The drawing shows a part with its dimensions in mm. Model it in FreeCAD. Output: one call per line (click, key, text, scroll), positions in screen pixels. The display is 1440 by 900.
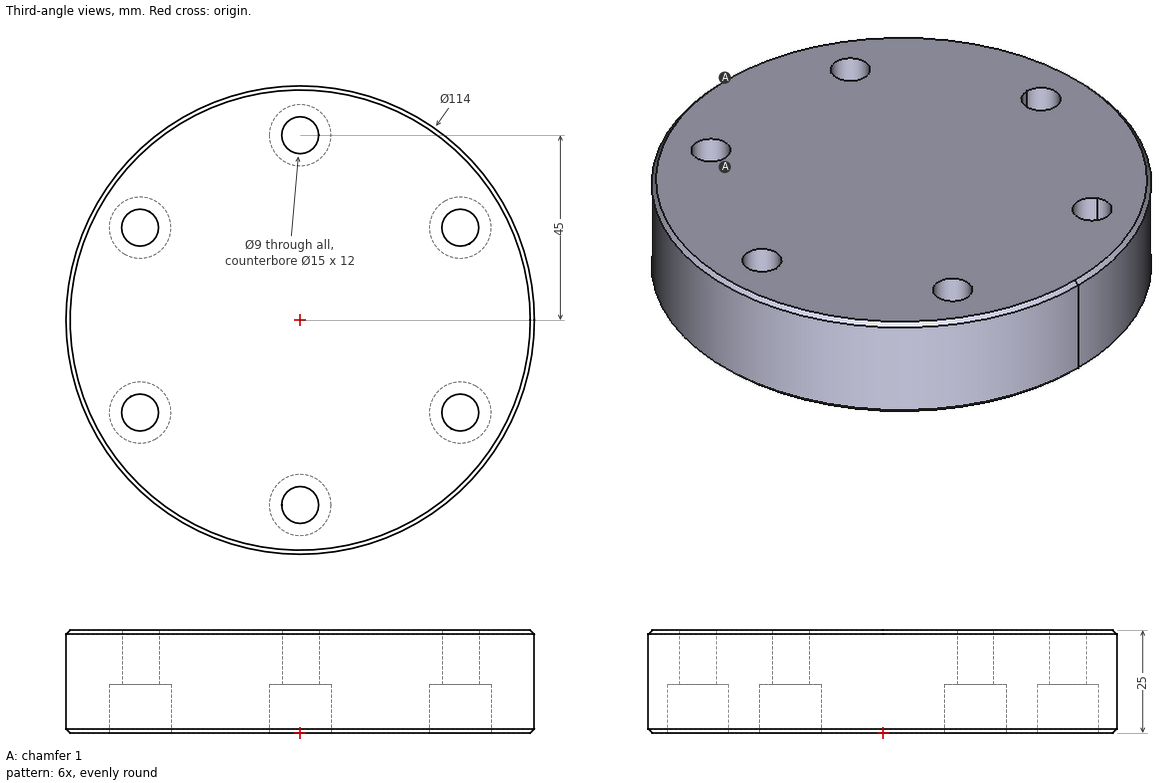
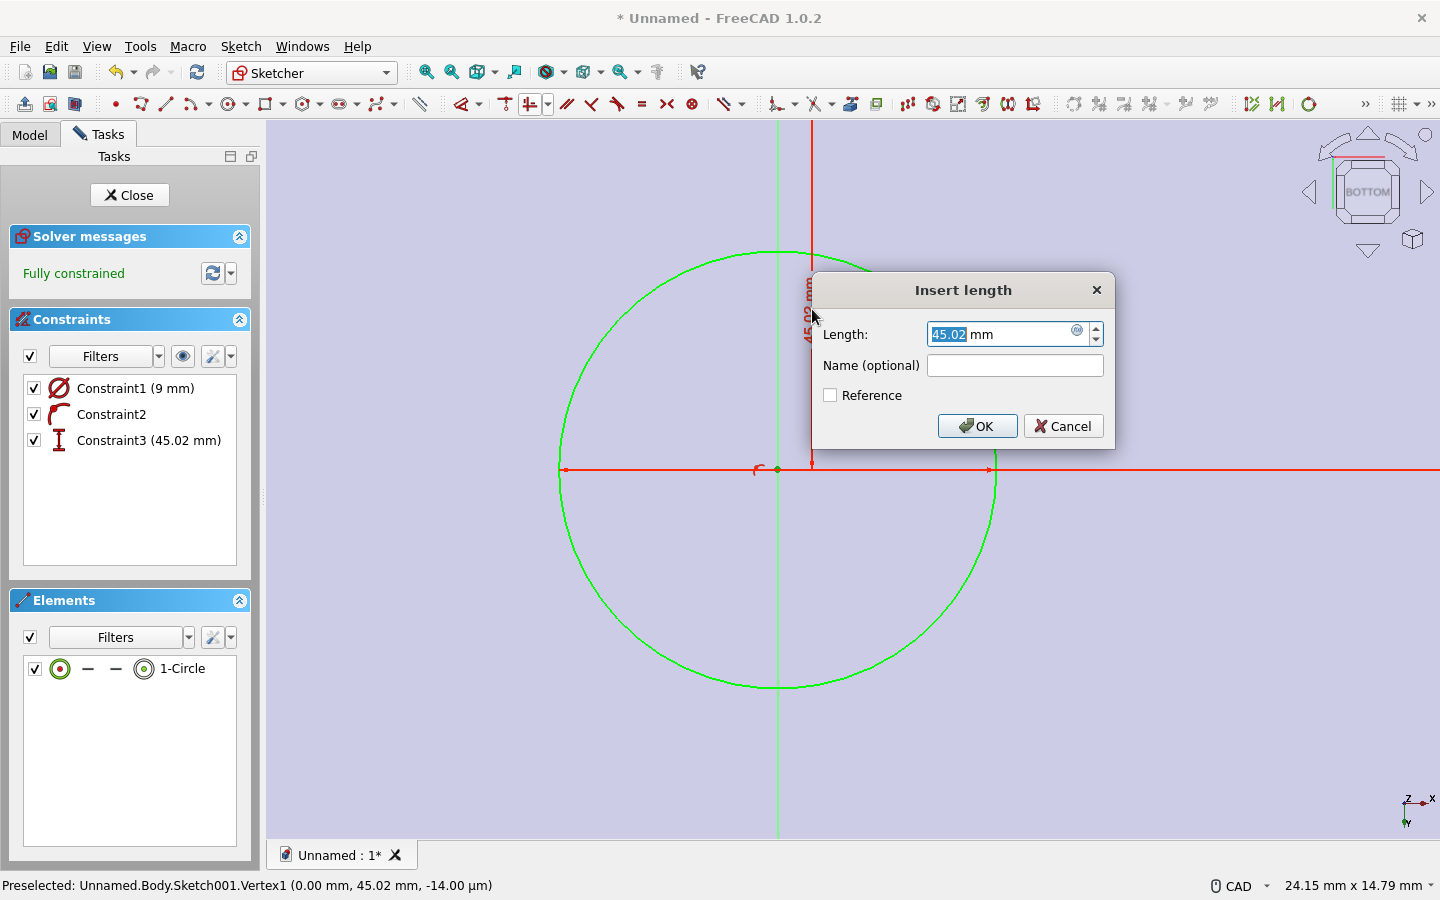
text(45)
key(Return)
key(Escape)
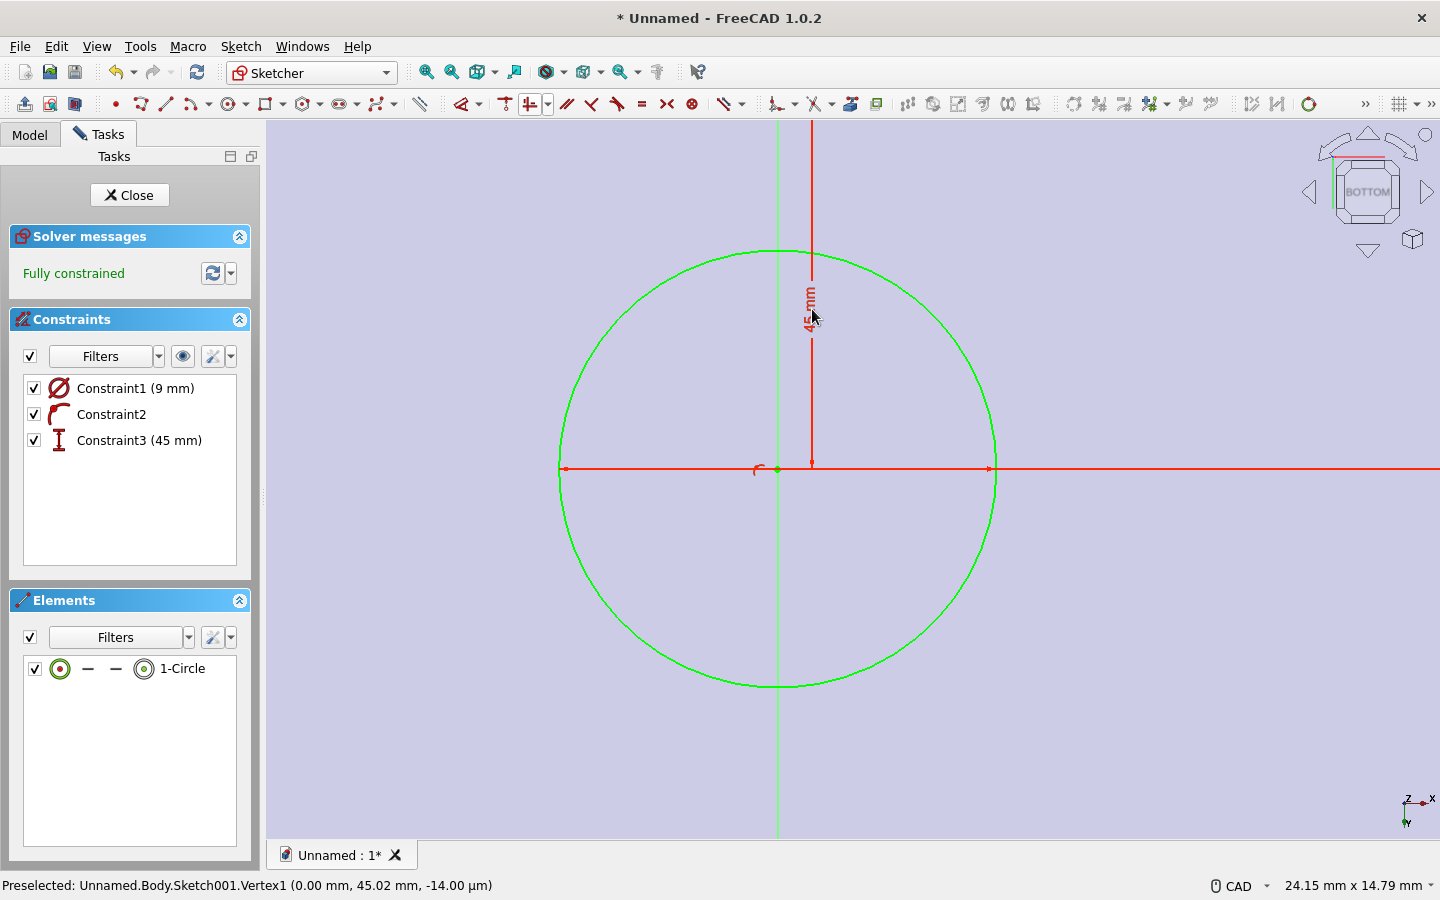
click(130, 195)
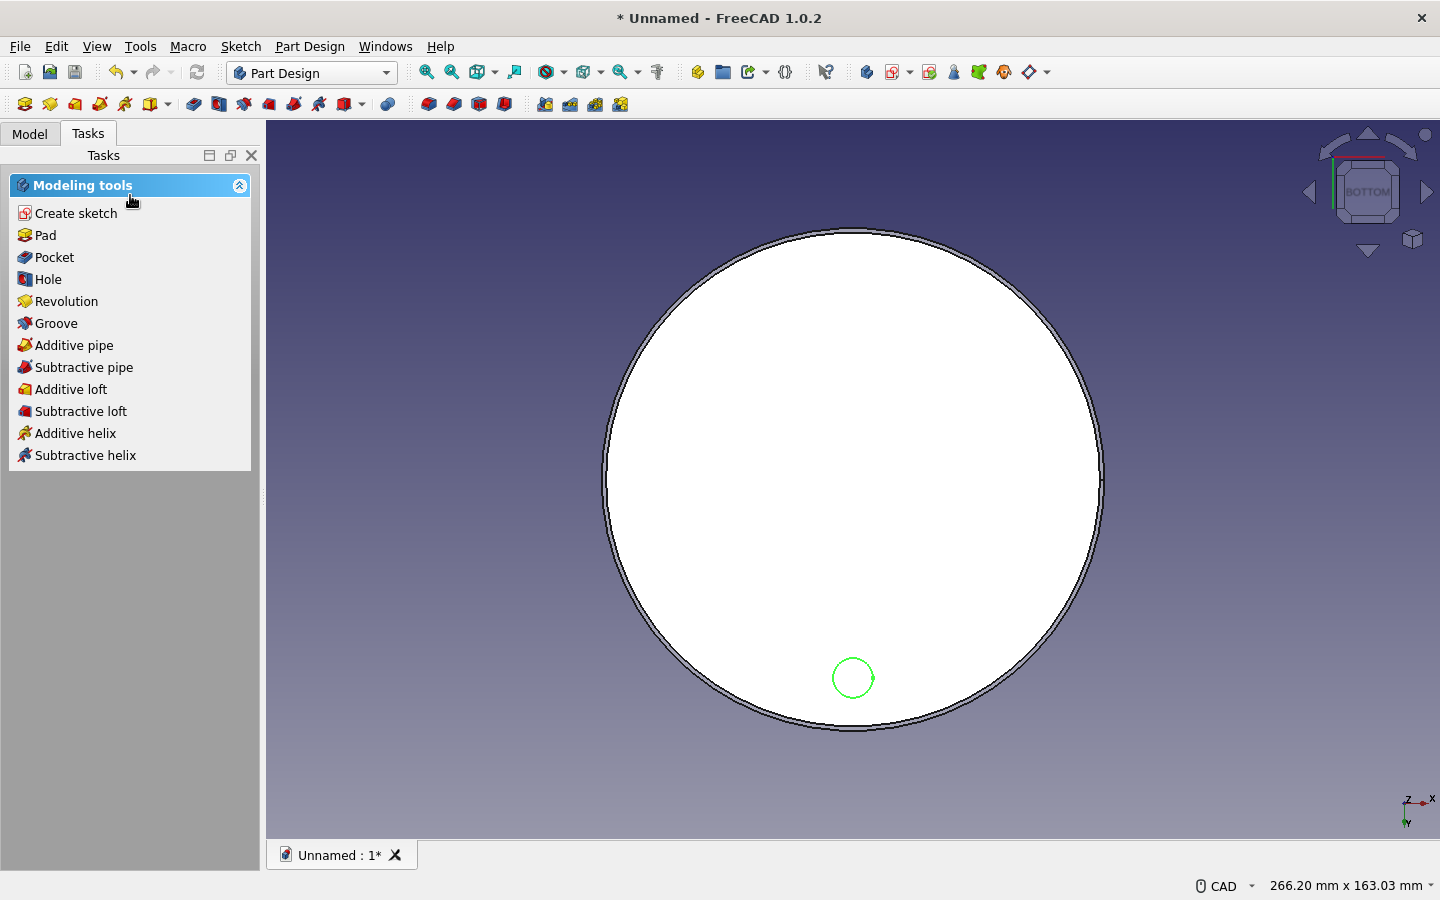
click(219, 104)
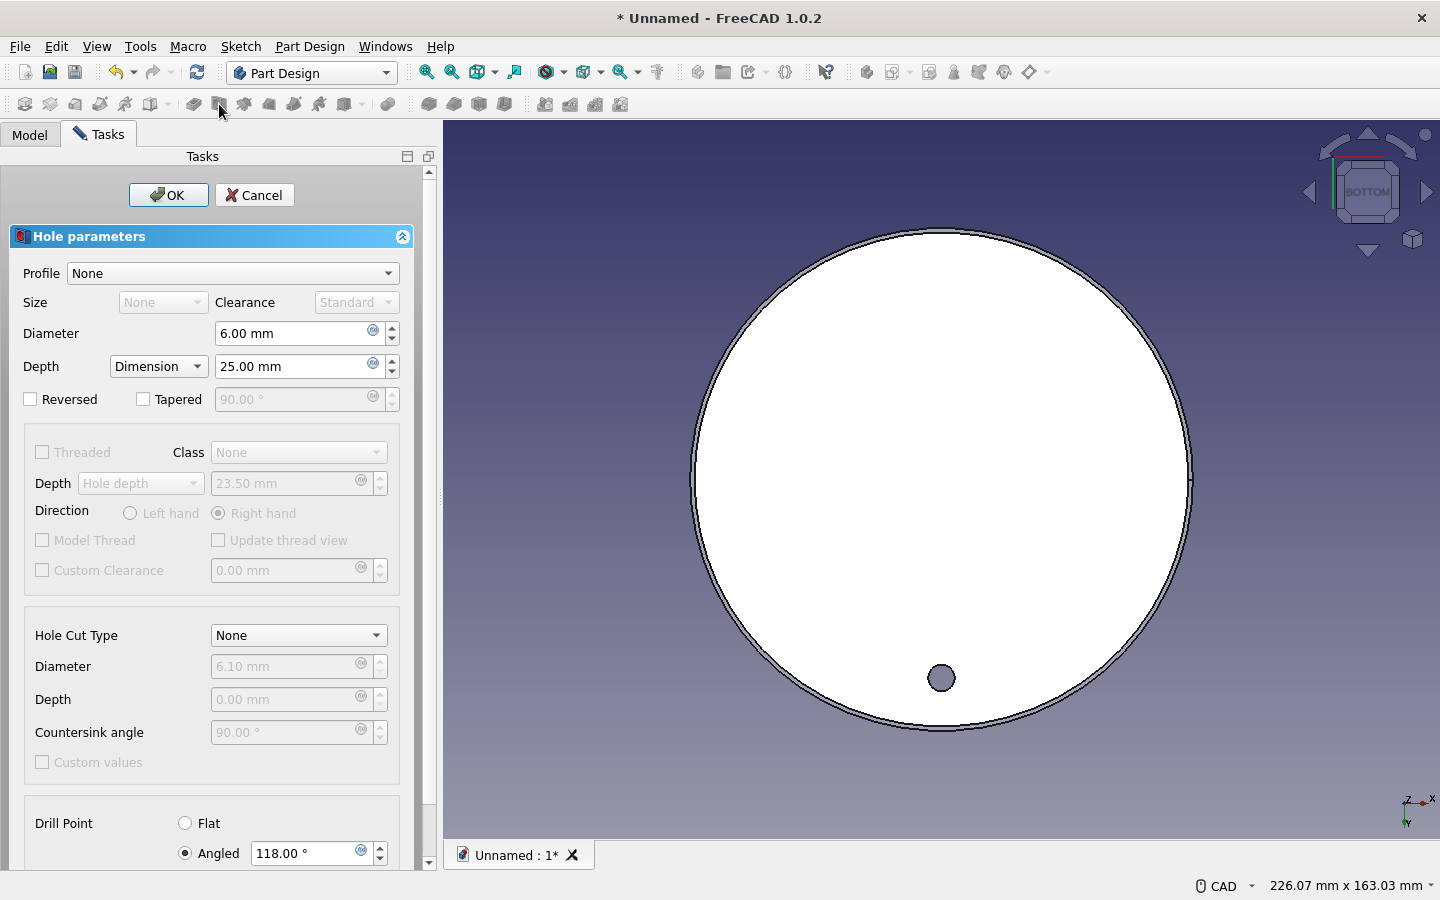
triple_click(300, 334)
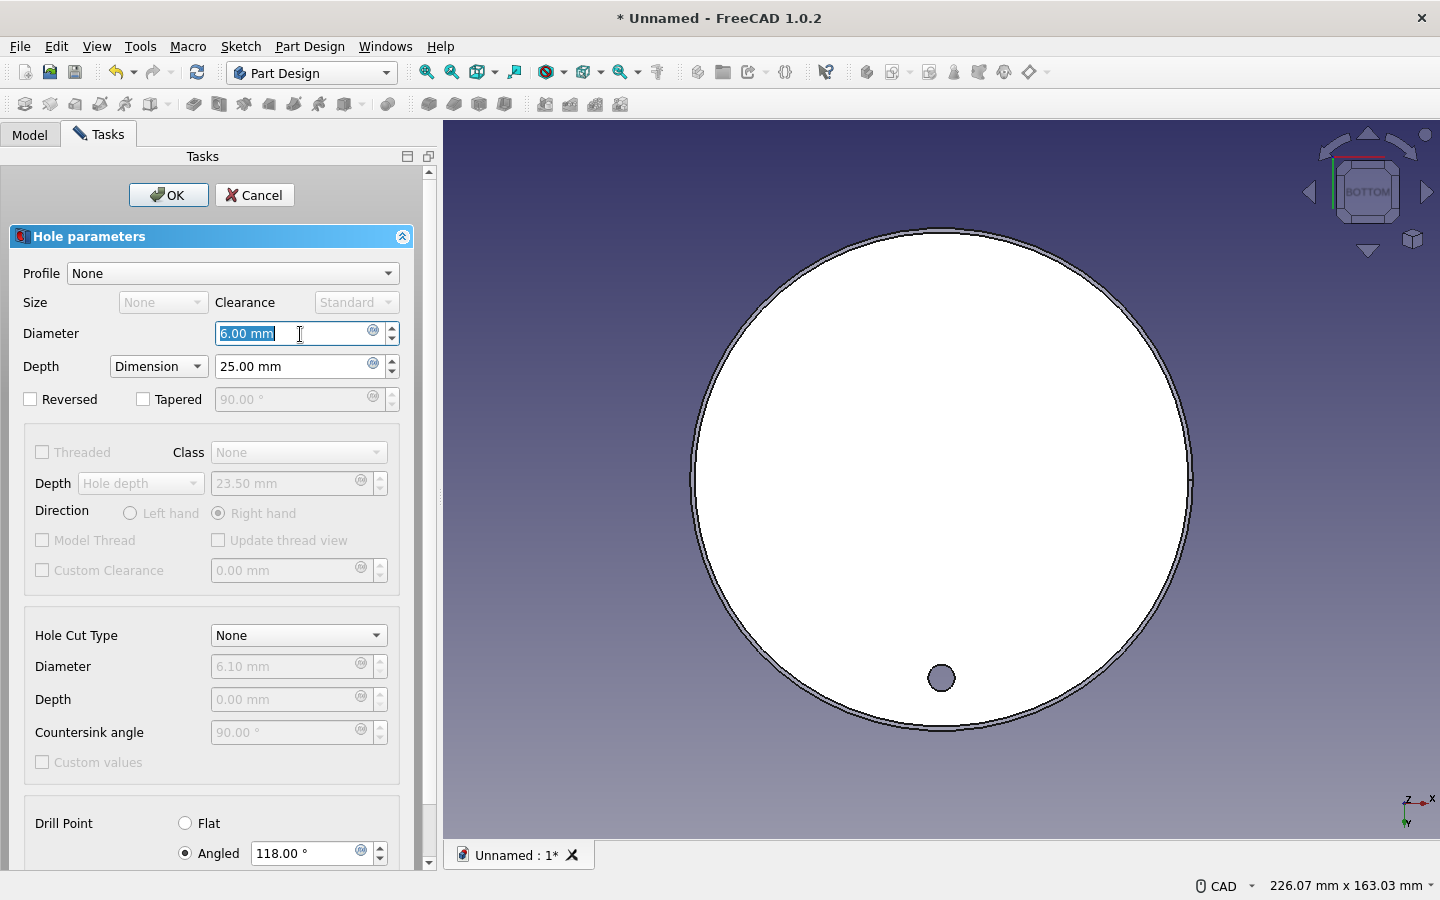
text(9)
key(Tab)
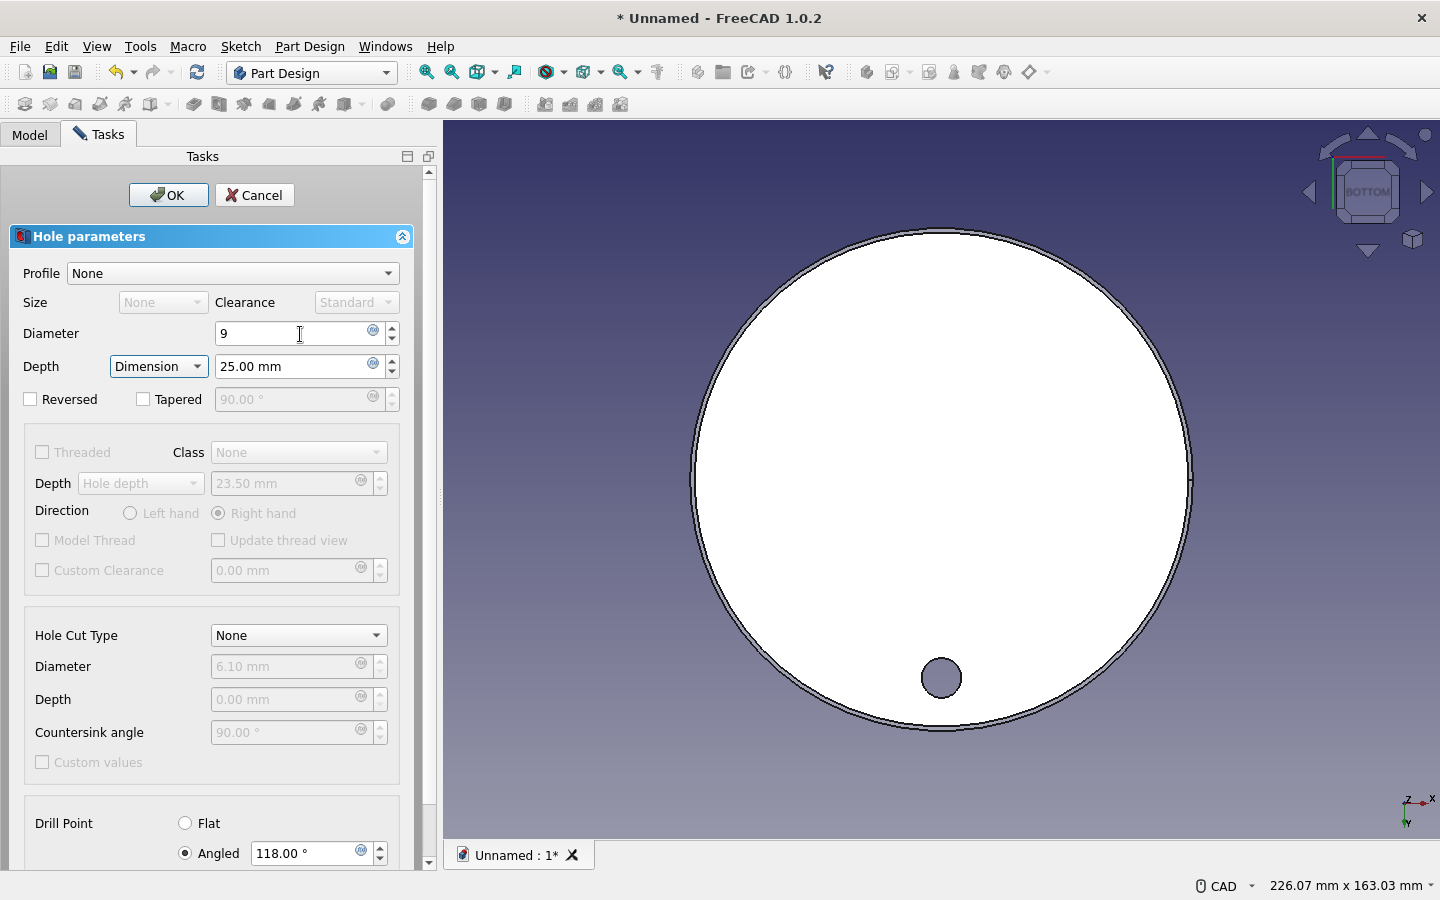
click(160, 366)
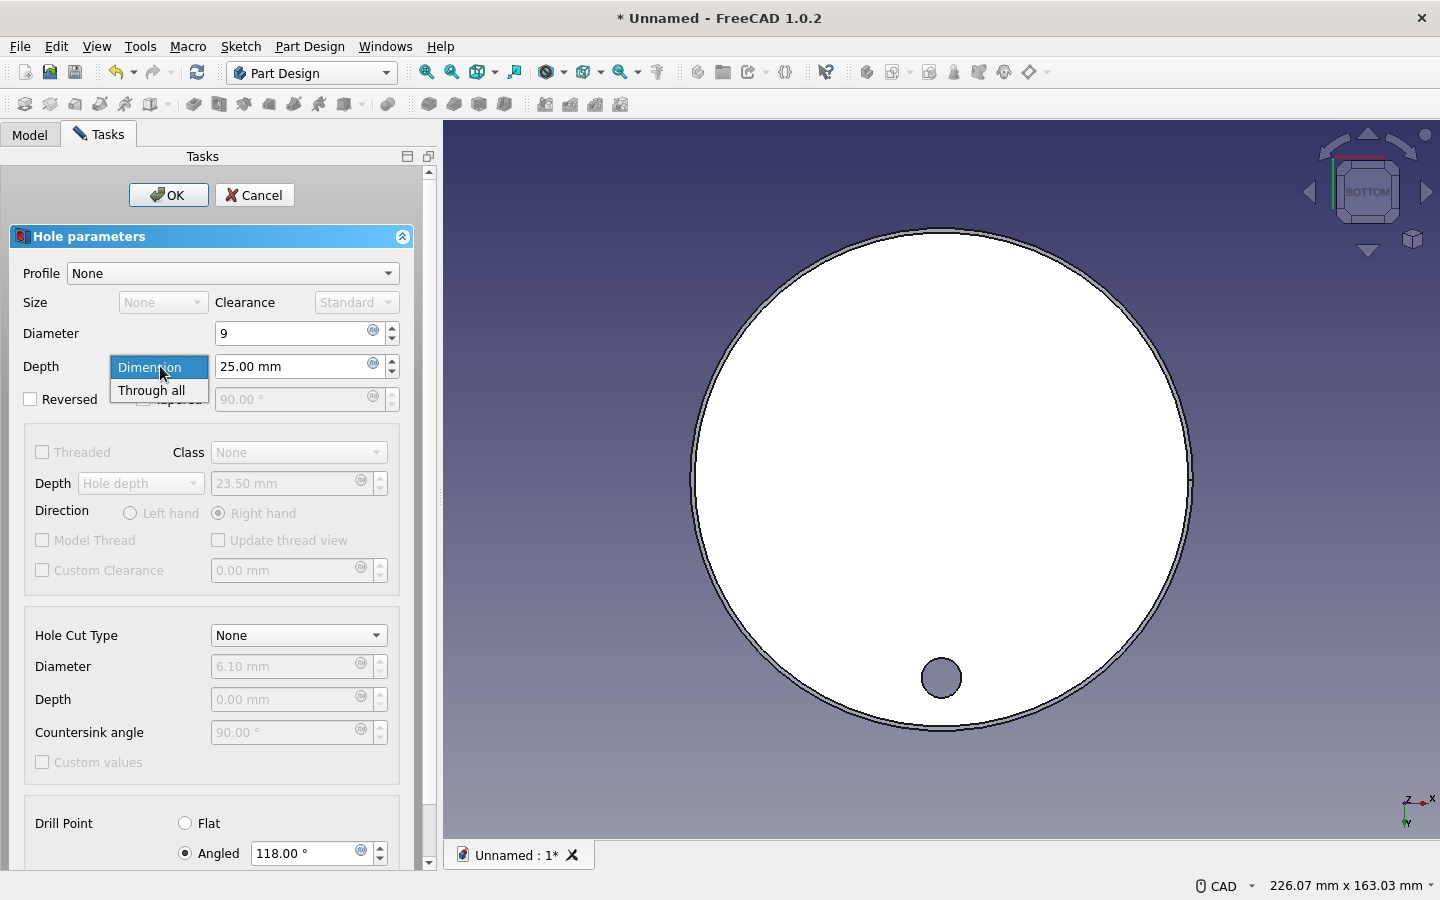
click(158, 390)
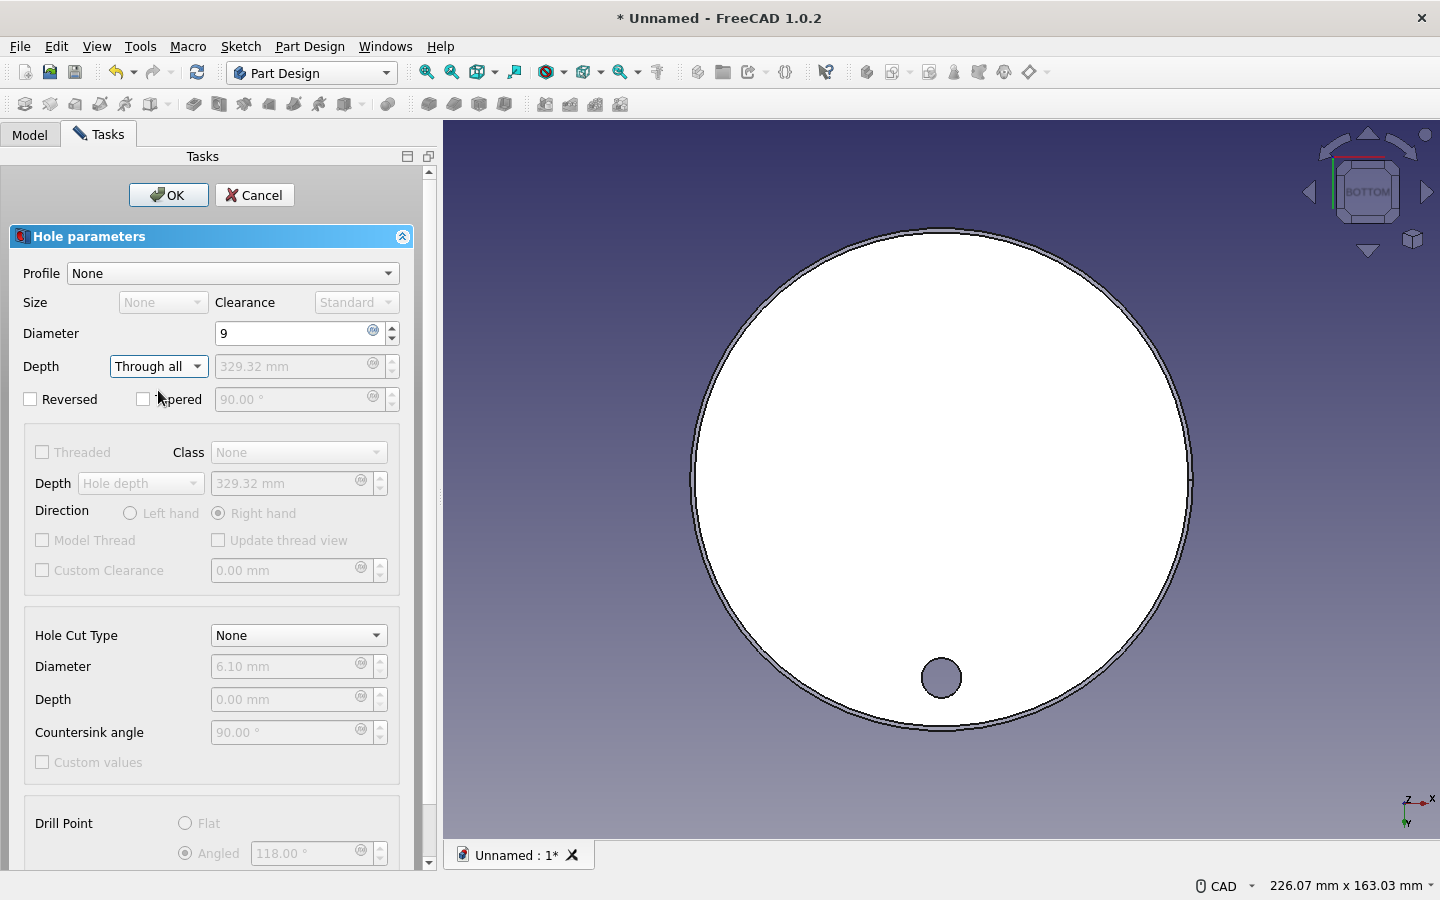
click(300, 636)